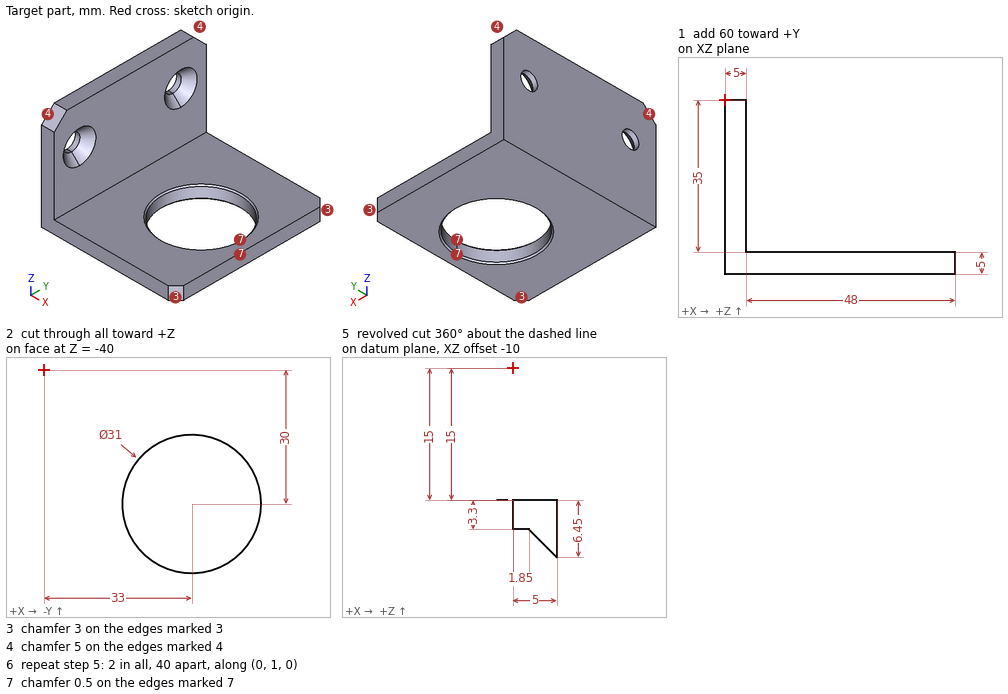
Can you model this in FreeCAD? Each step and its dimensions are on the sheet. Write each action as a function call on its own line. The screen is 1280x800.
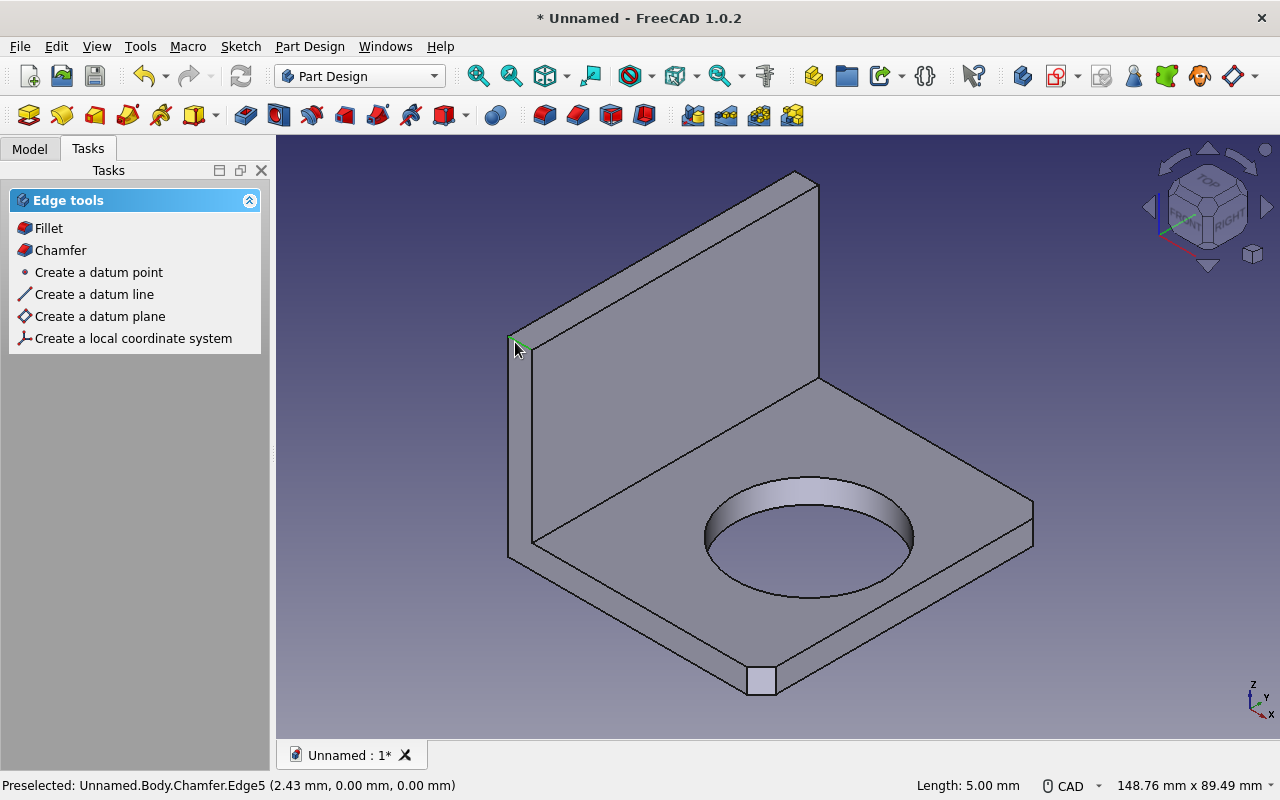
key(2)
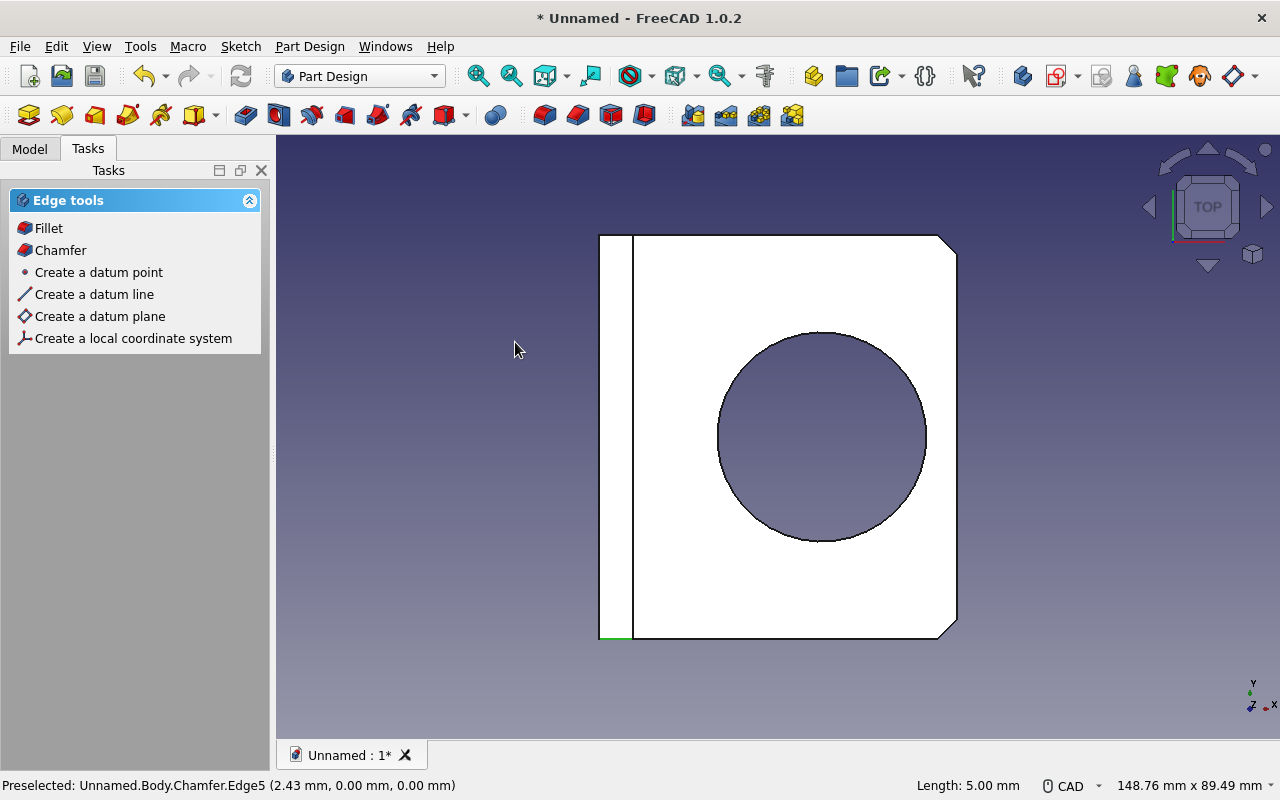
click(616, 234, ctrl)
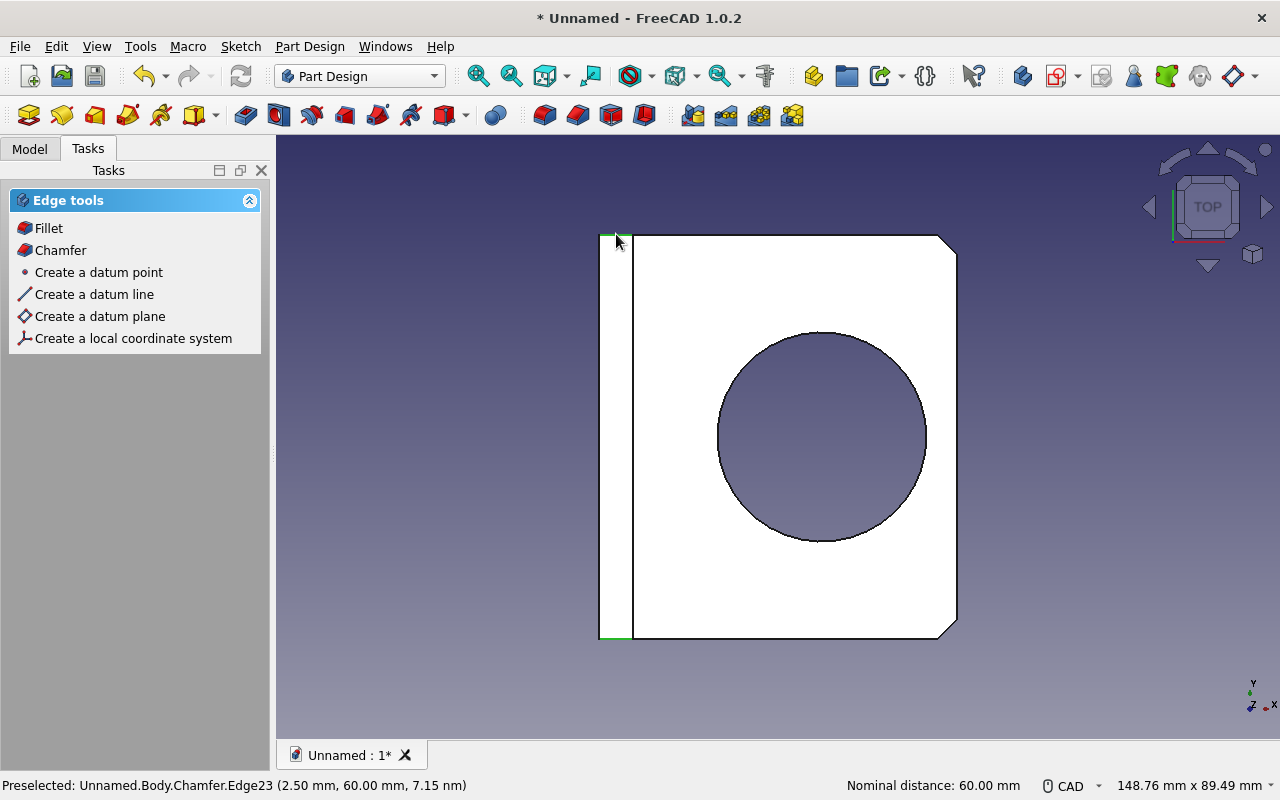
click(578, 116)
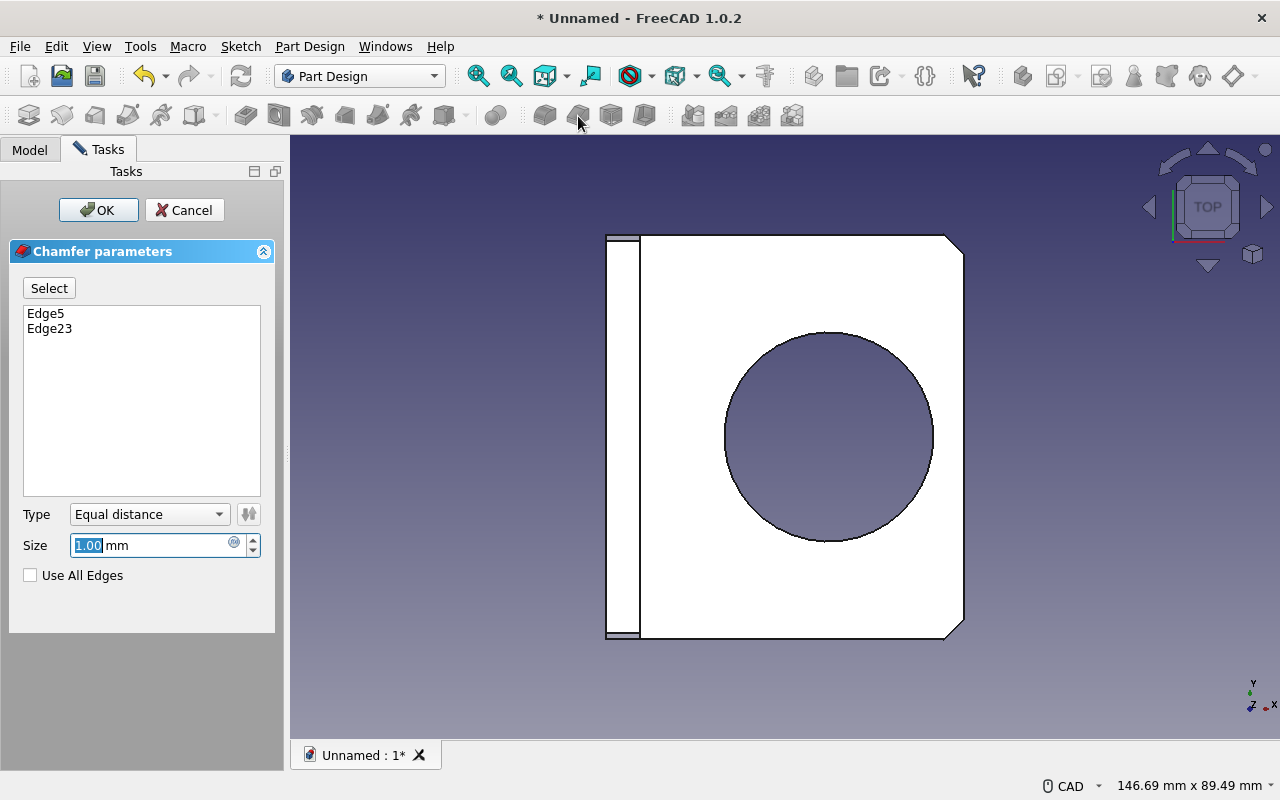
text(5)
key(Tab)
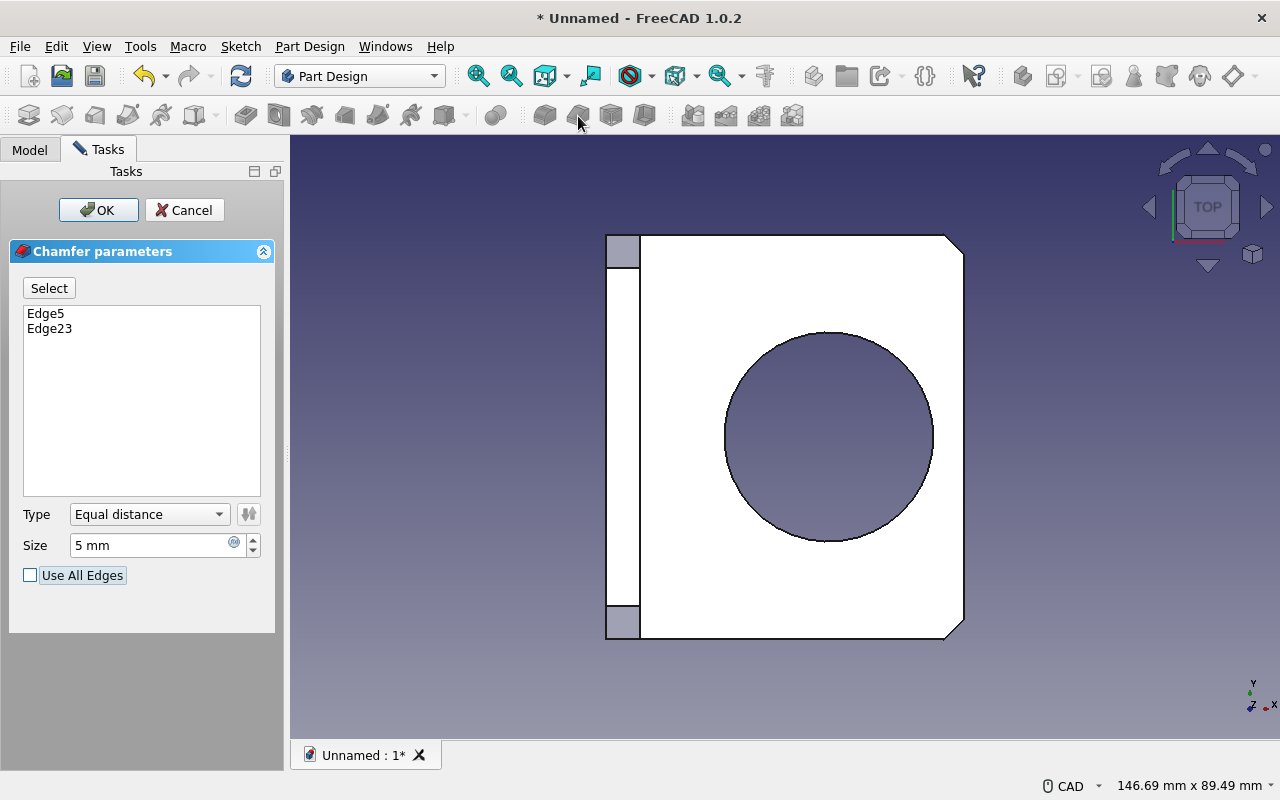
click(99, 210)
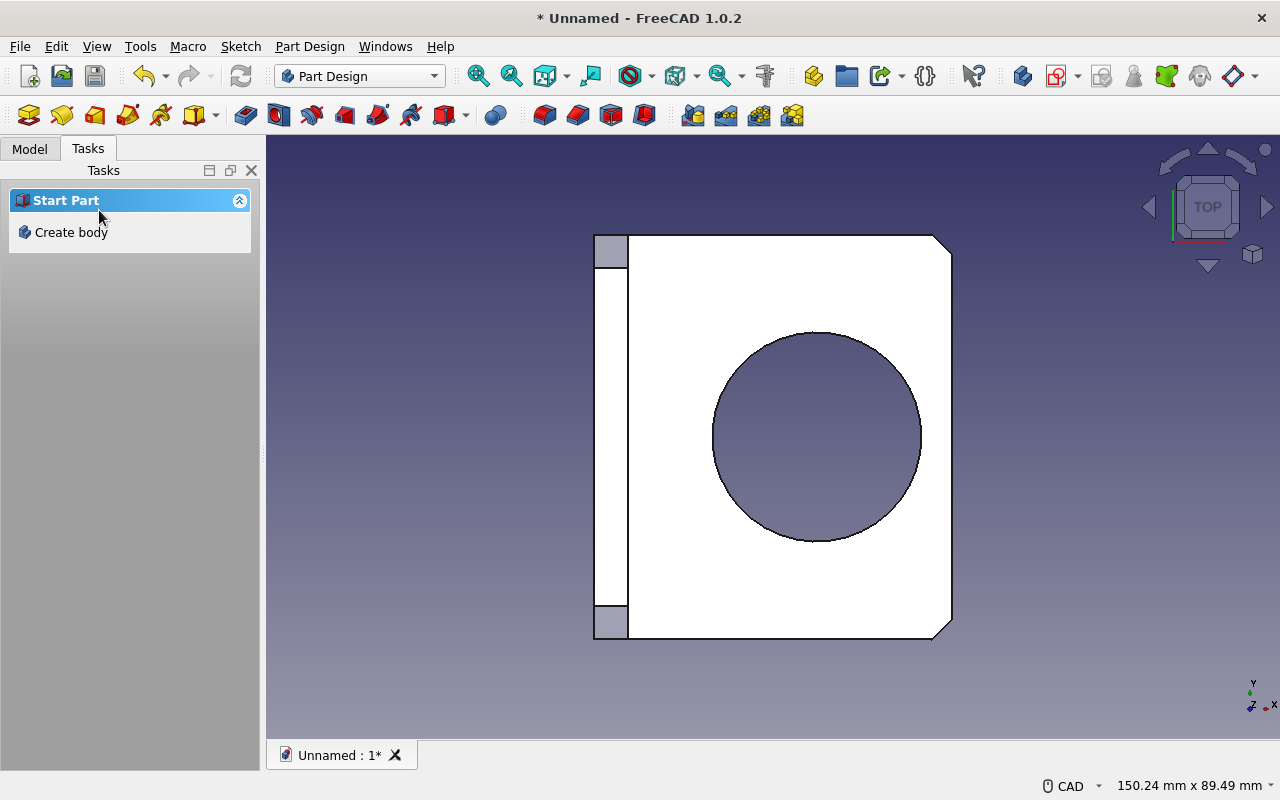
click(30, 148)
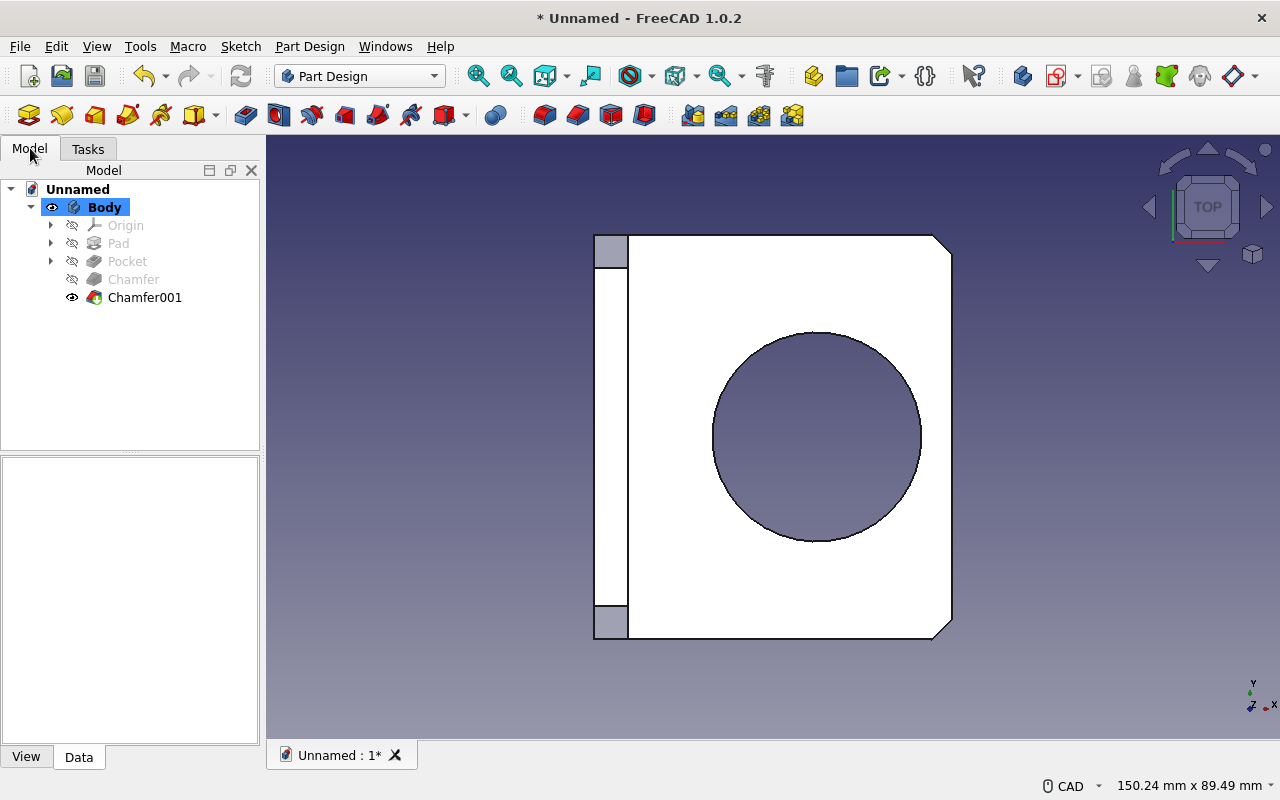
click(51, 225)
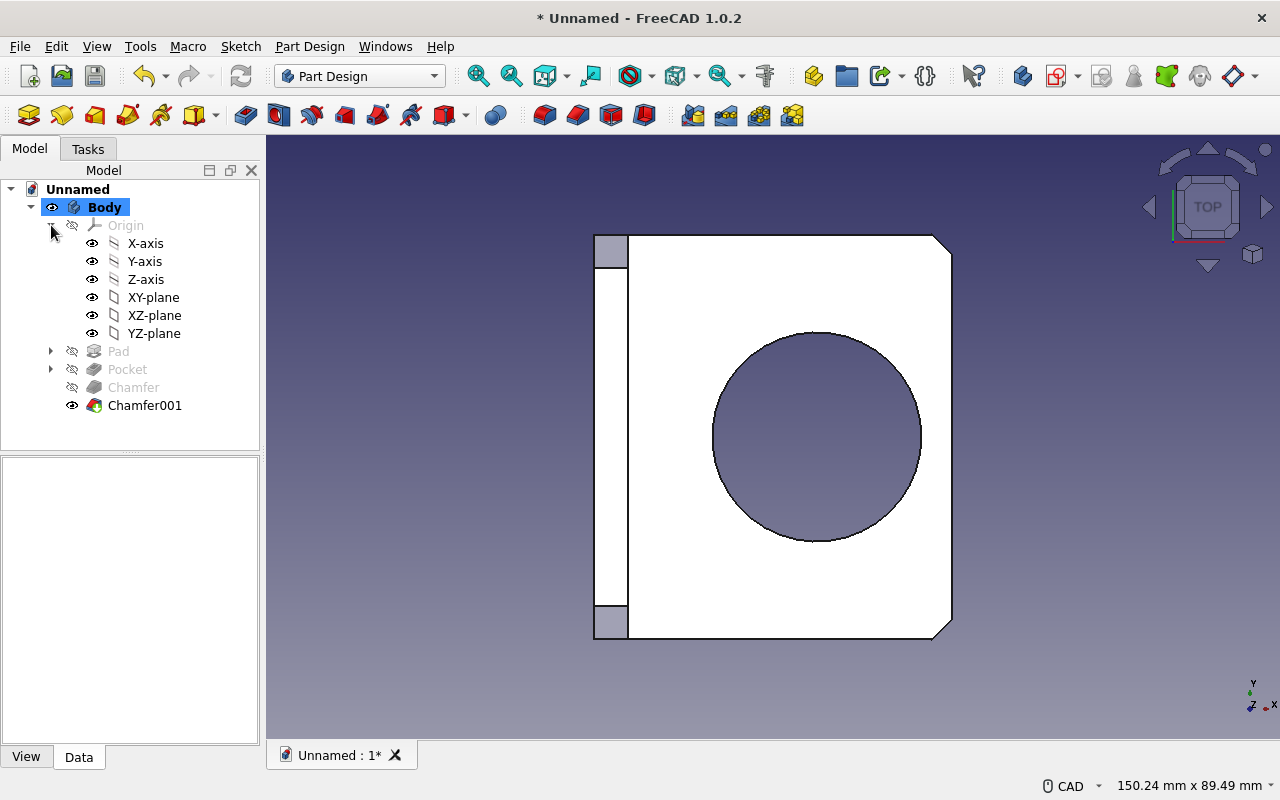
click(137, 315)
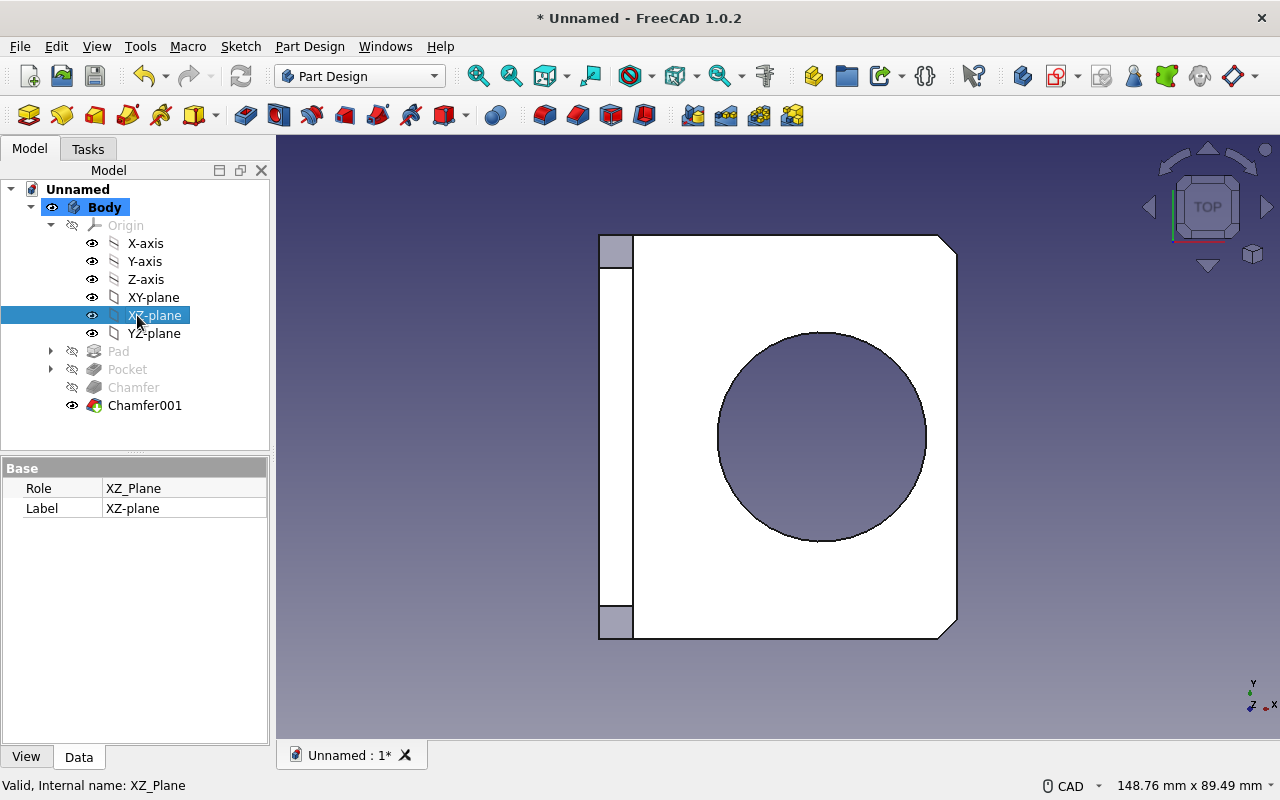
click(1232, 76)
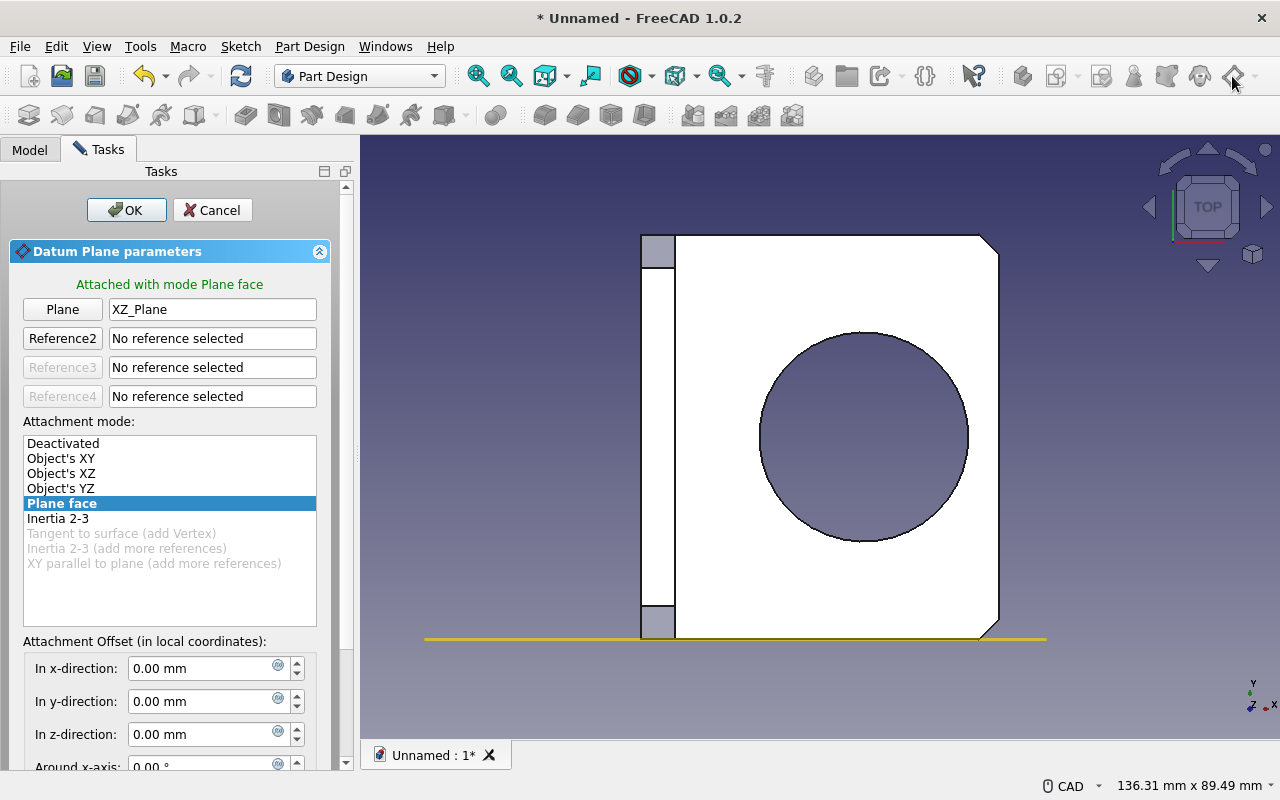
triple_click(210, 734)